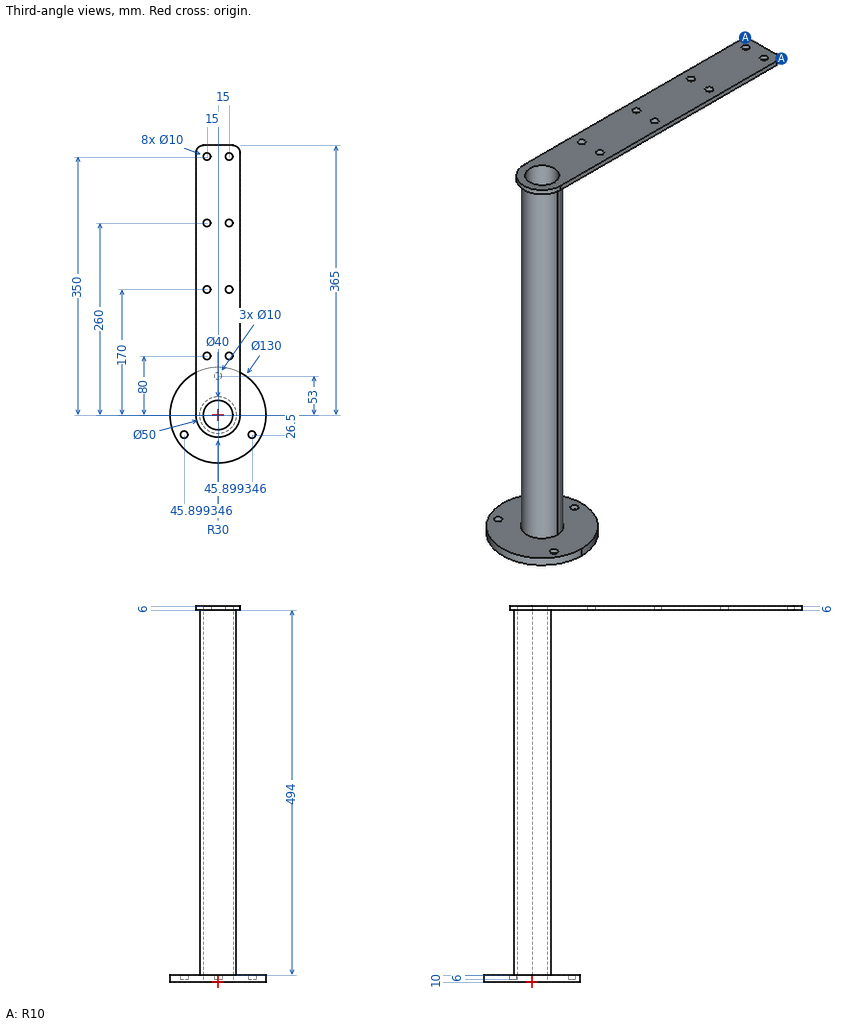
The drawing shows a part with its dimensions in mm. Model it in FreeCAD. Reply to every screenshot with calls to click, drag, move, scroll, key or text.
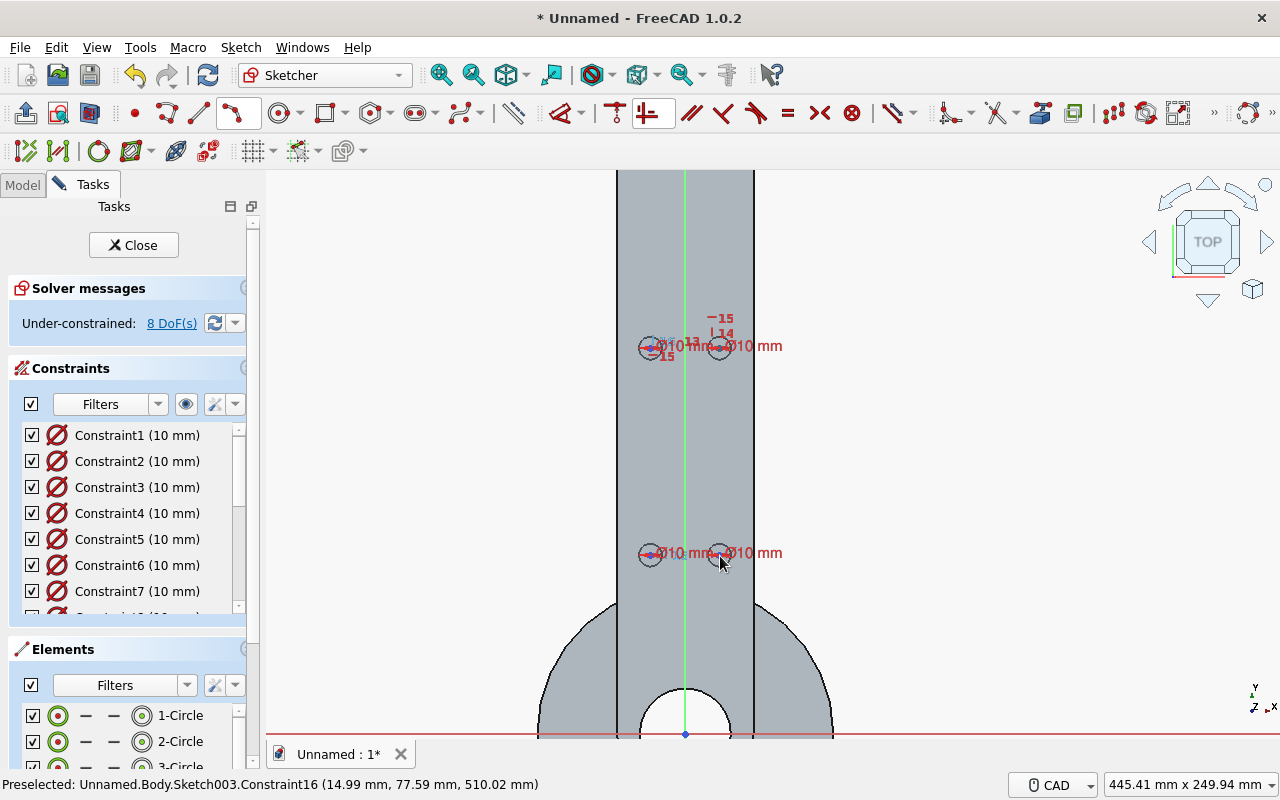
click(719, 555)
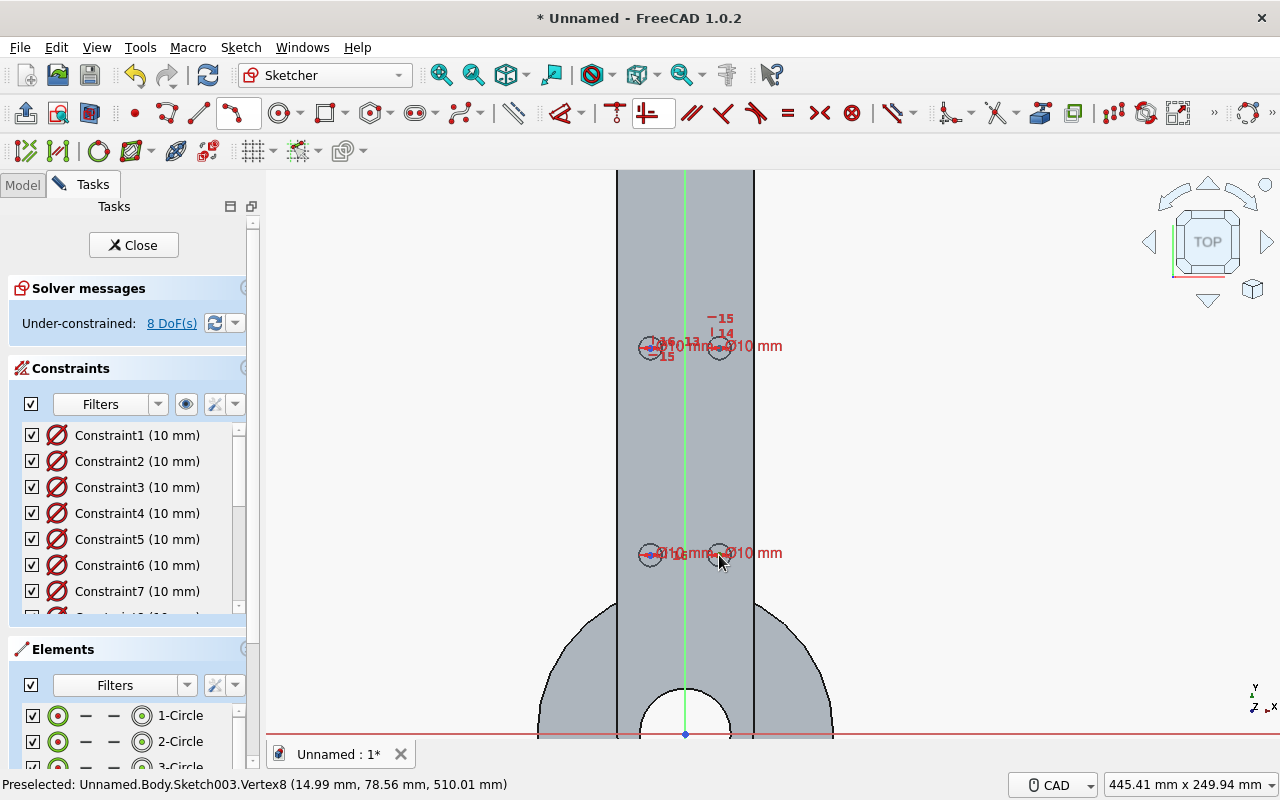
key(v)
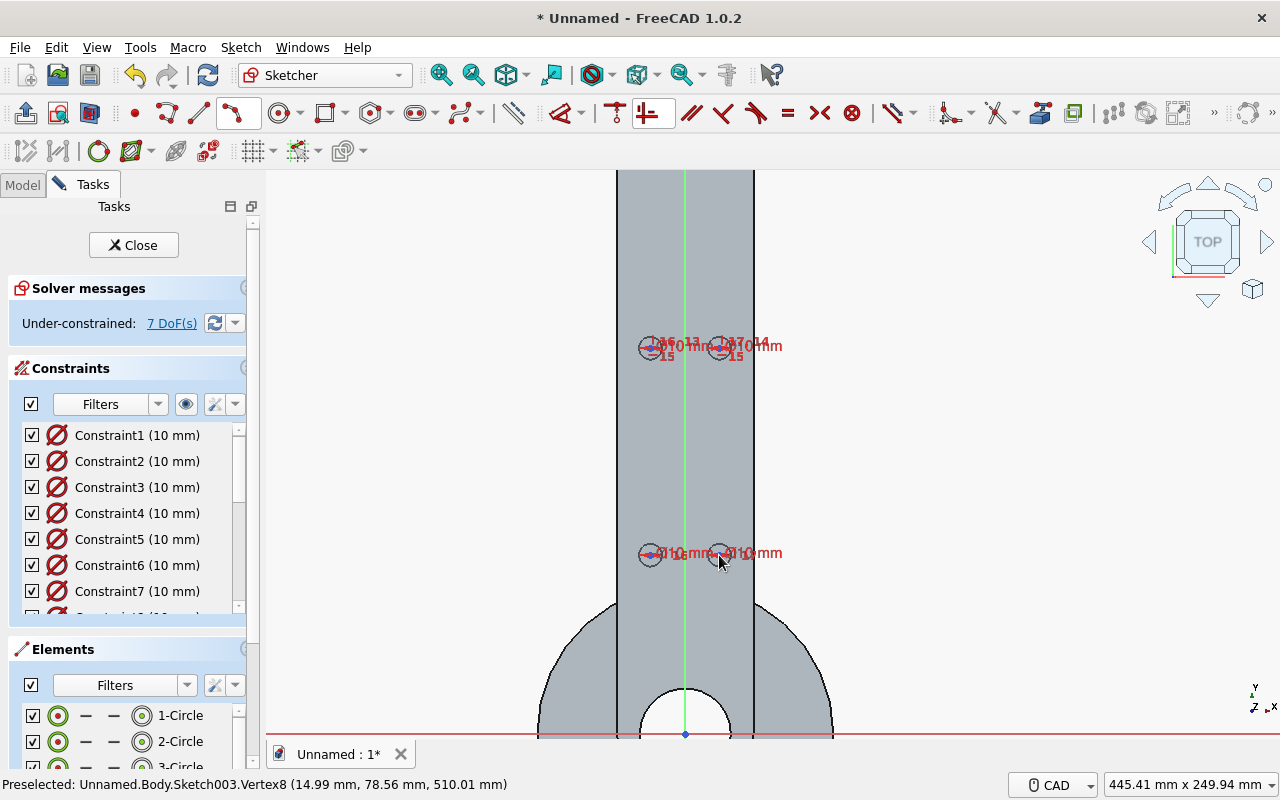
click(650, 555)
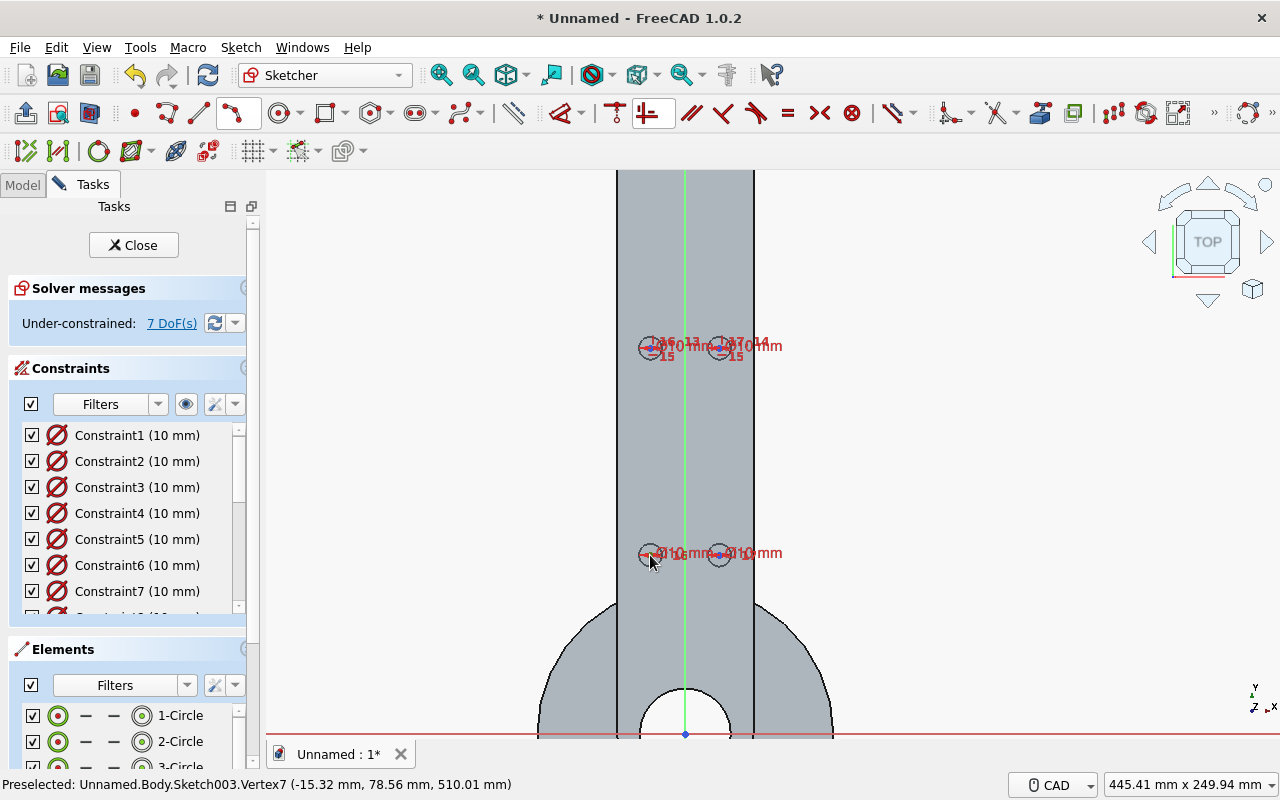
click(719, 555)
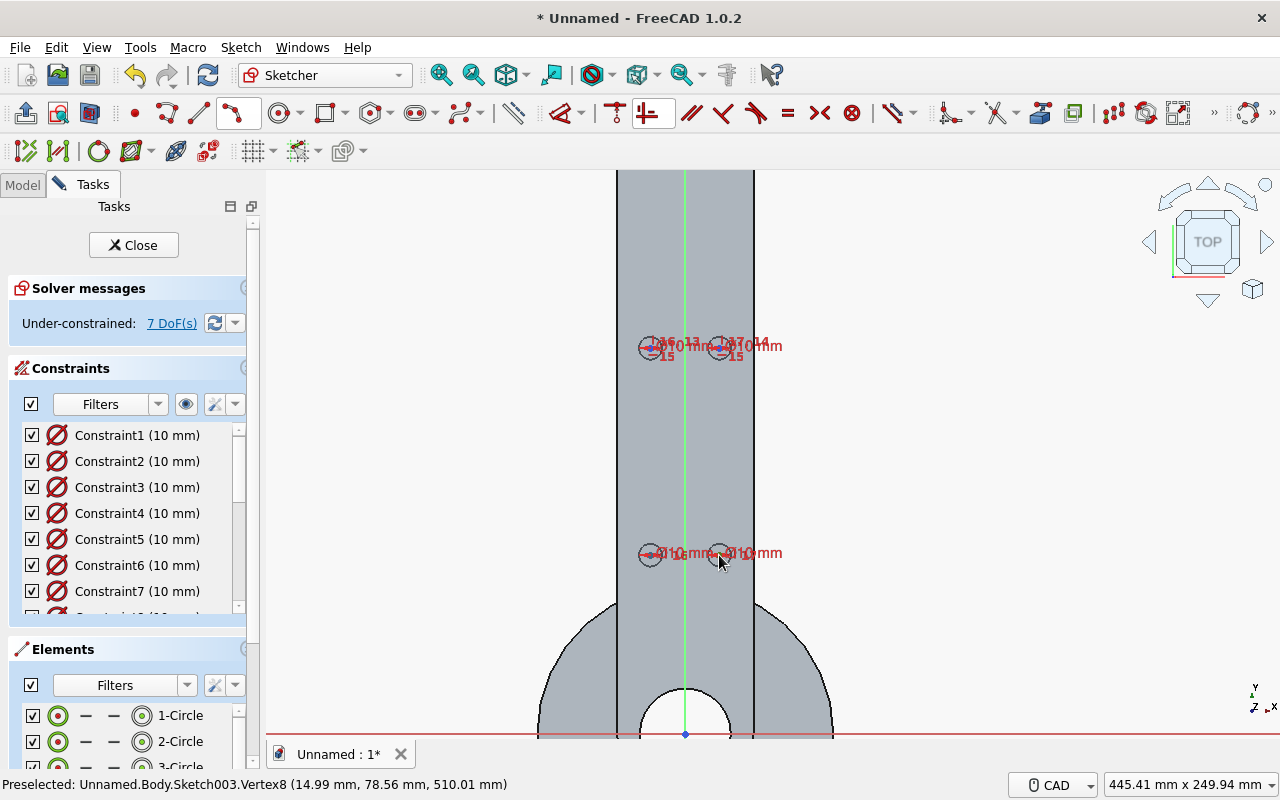
click(670, 114)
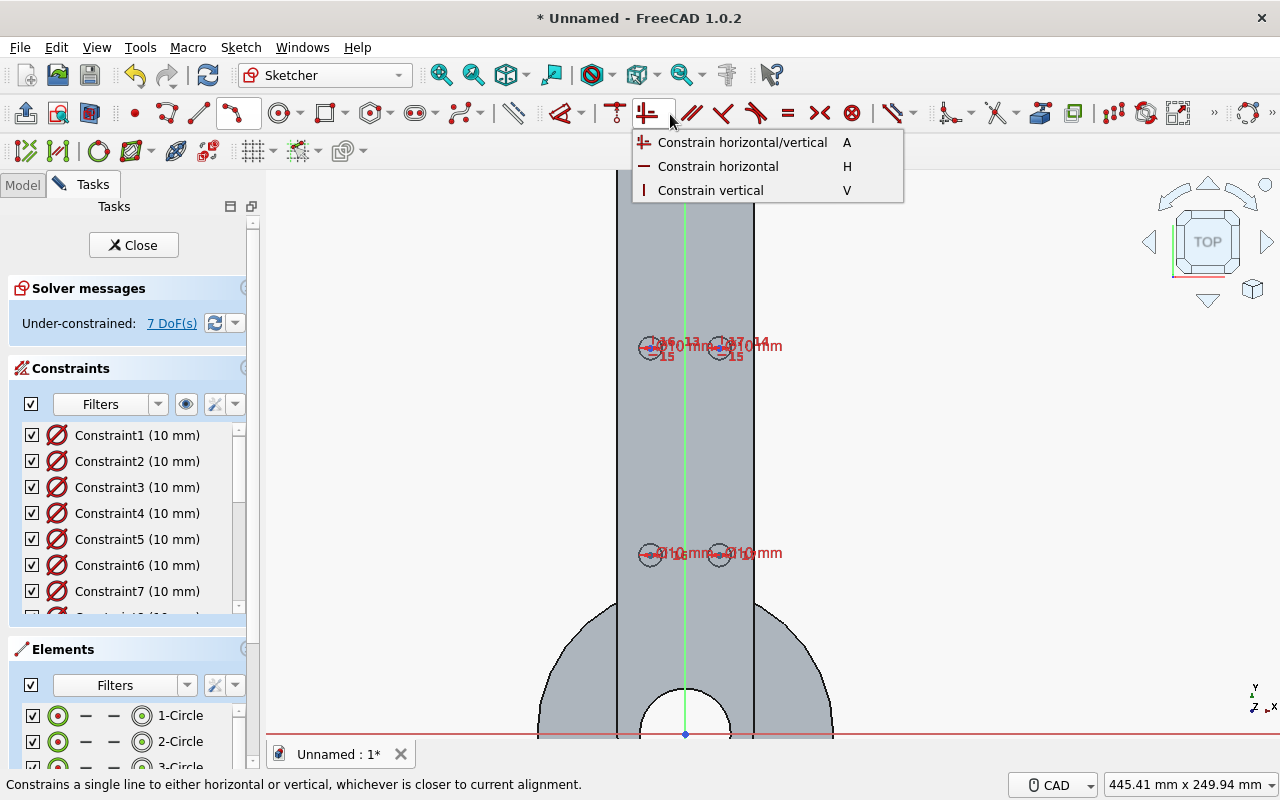
click(768, 166)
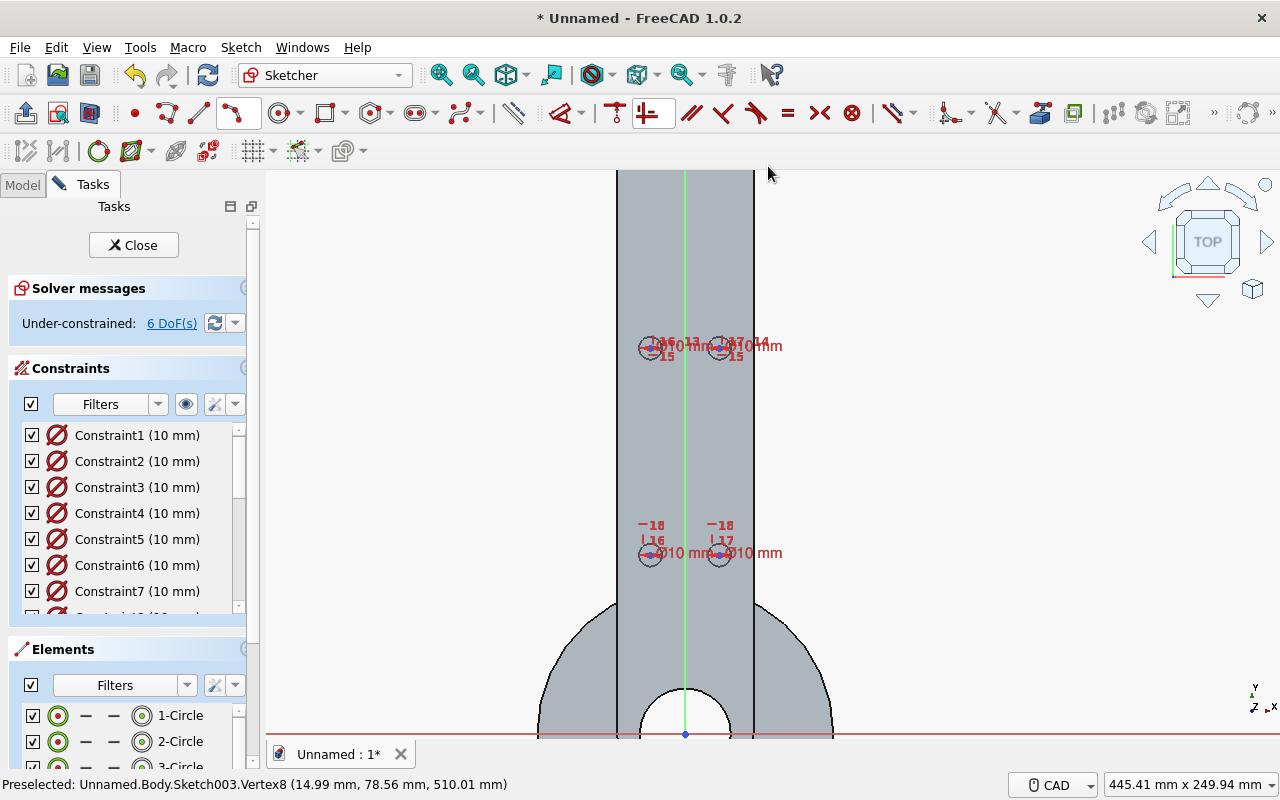
click(560, 114)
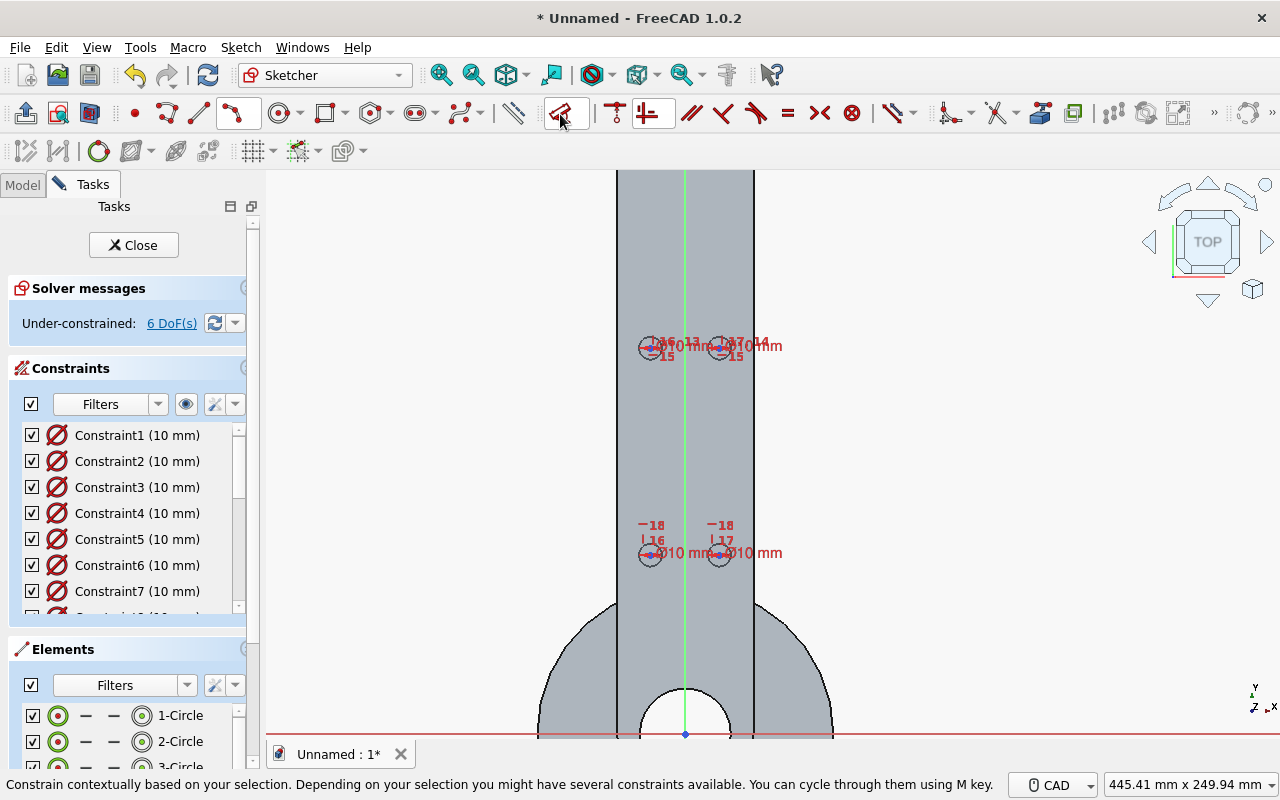
scroll(720, 556, down, 4)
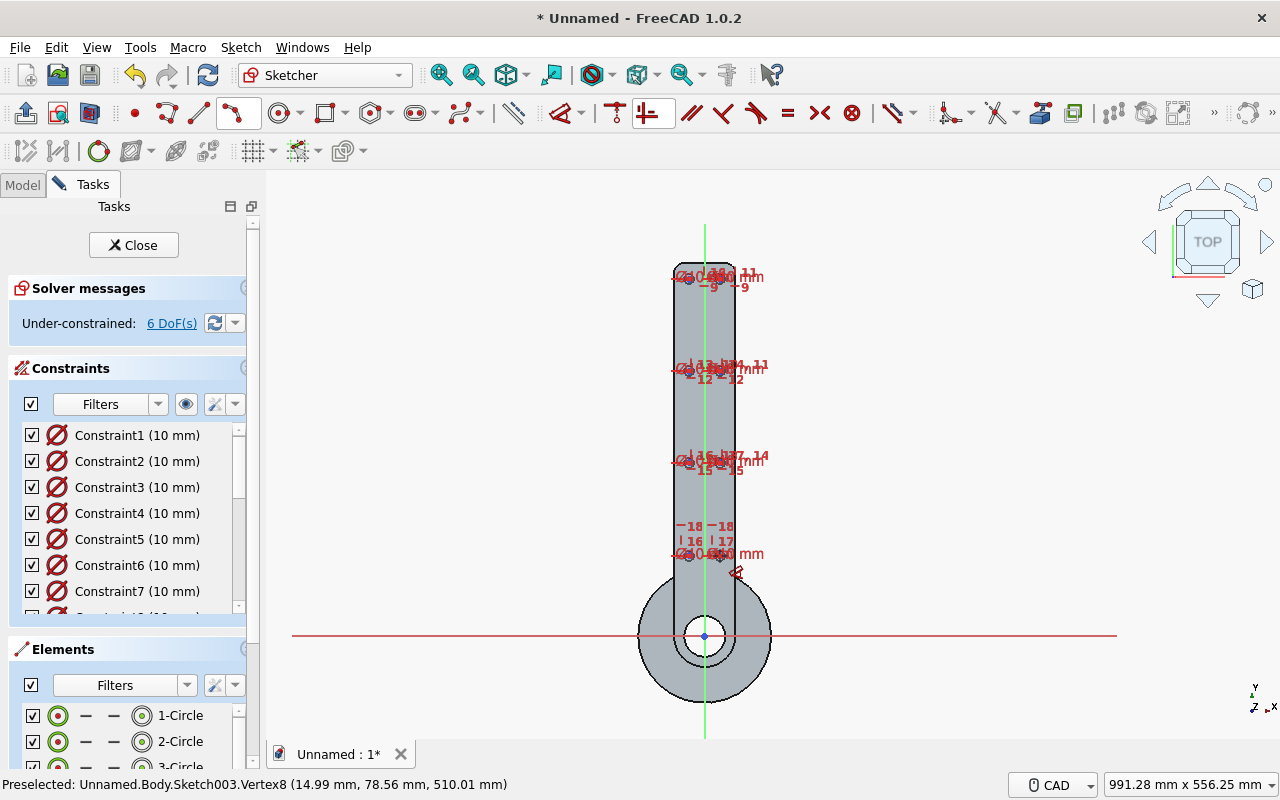
scroll(689, 279, up, 5)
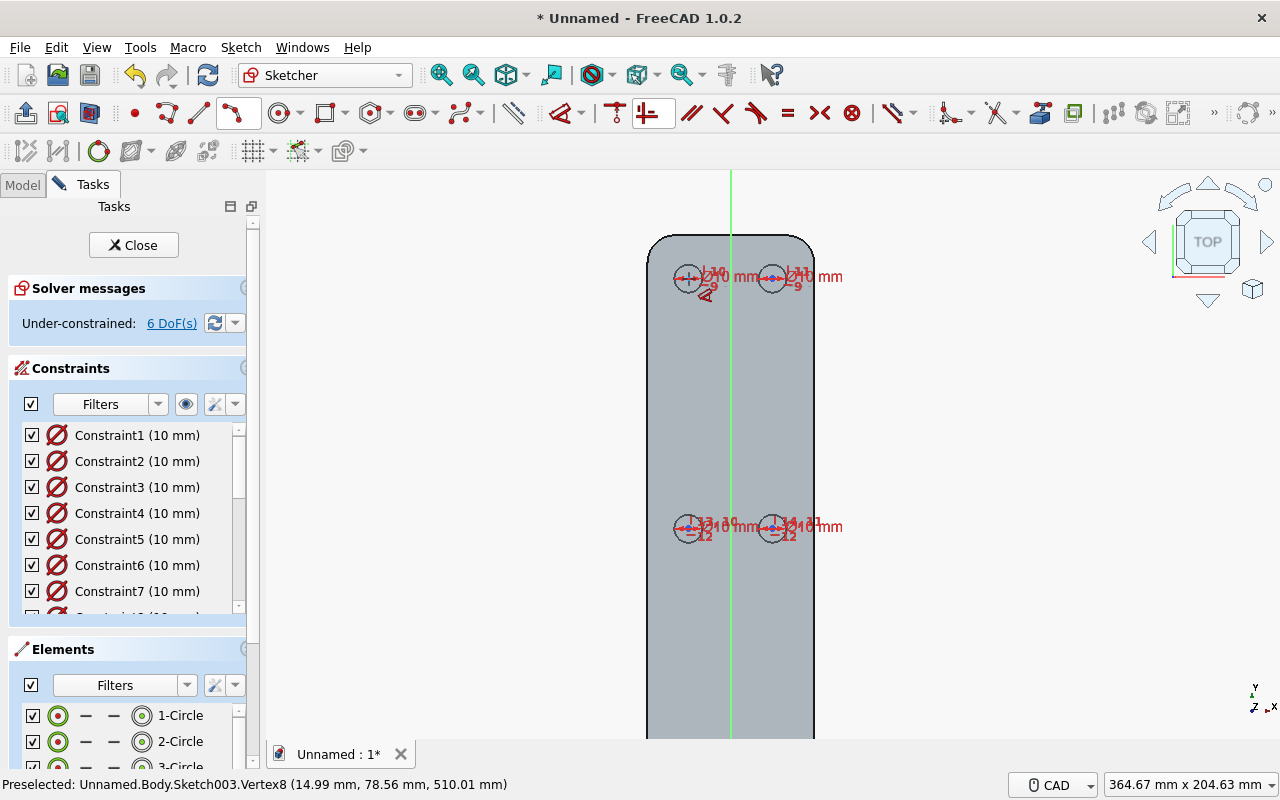
click(688, 279)
click(710, 245)